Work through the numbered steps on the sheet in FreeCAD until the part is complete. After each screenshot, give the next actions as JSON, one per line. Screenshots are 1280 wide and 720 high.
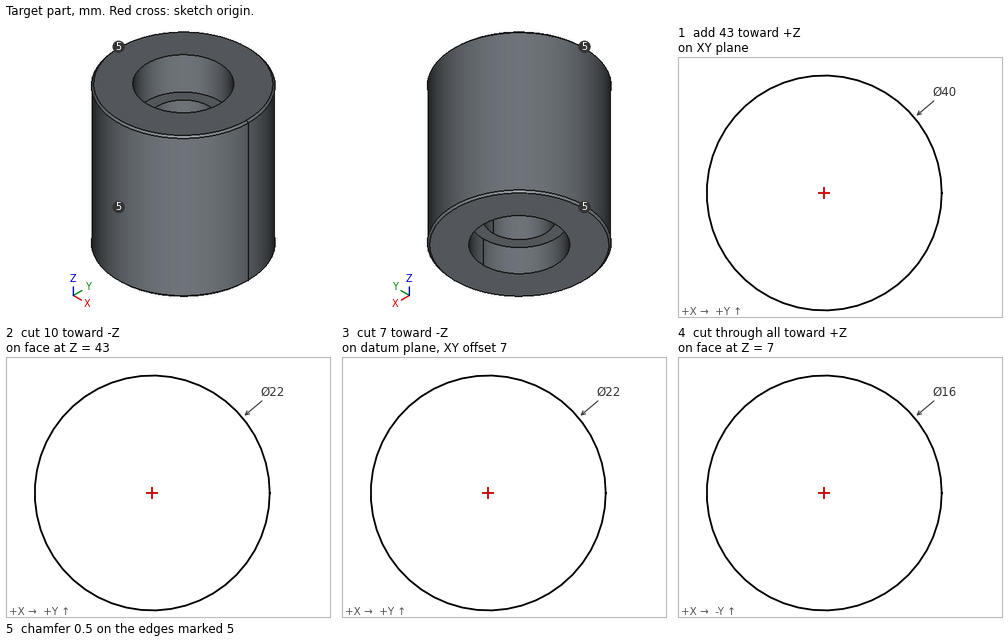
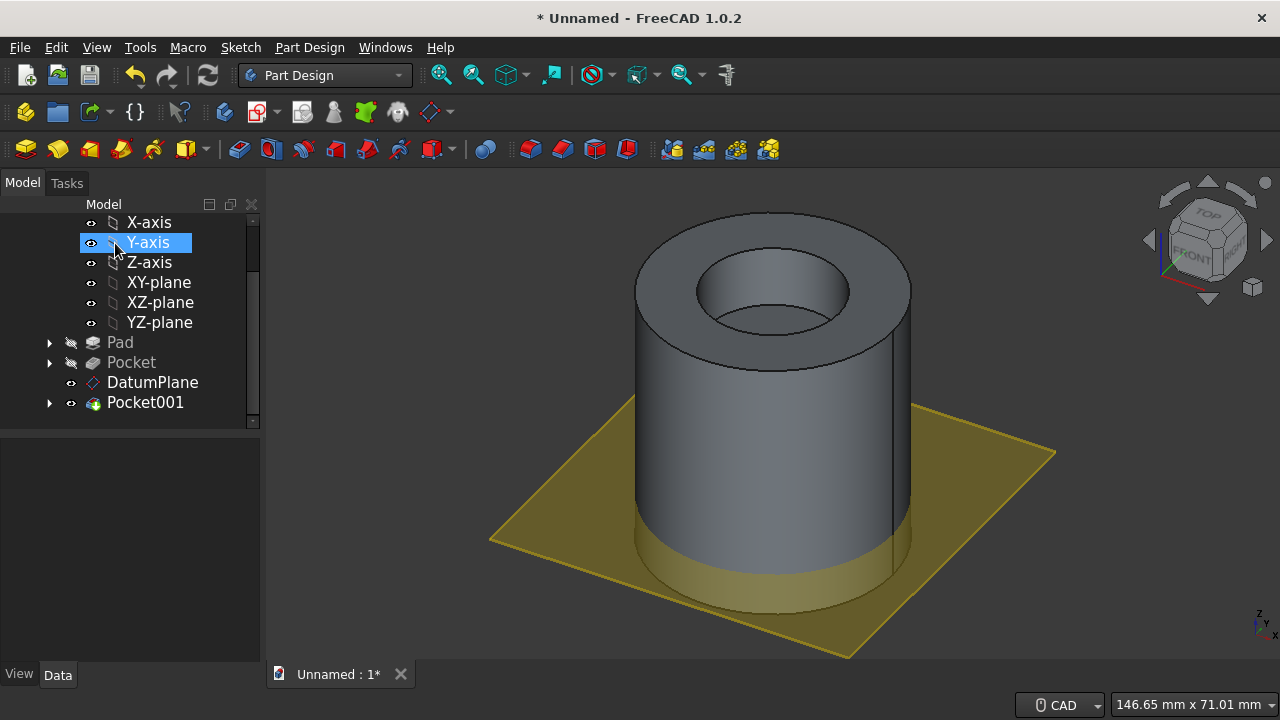
{"action": "left_click", "coordinate": [116, 383]}
{"action": "key", "text": "space"}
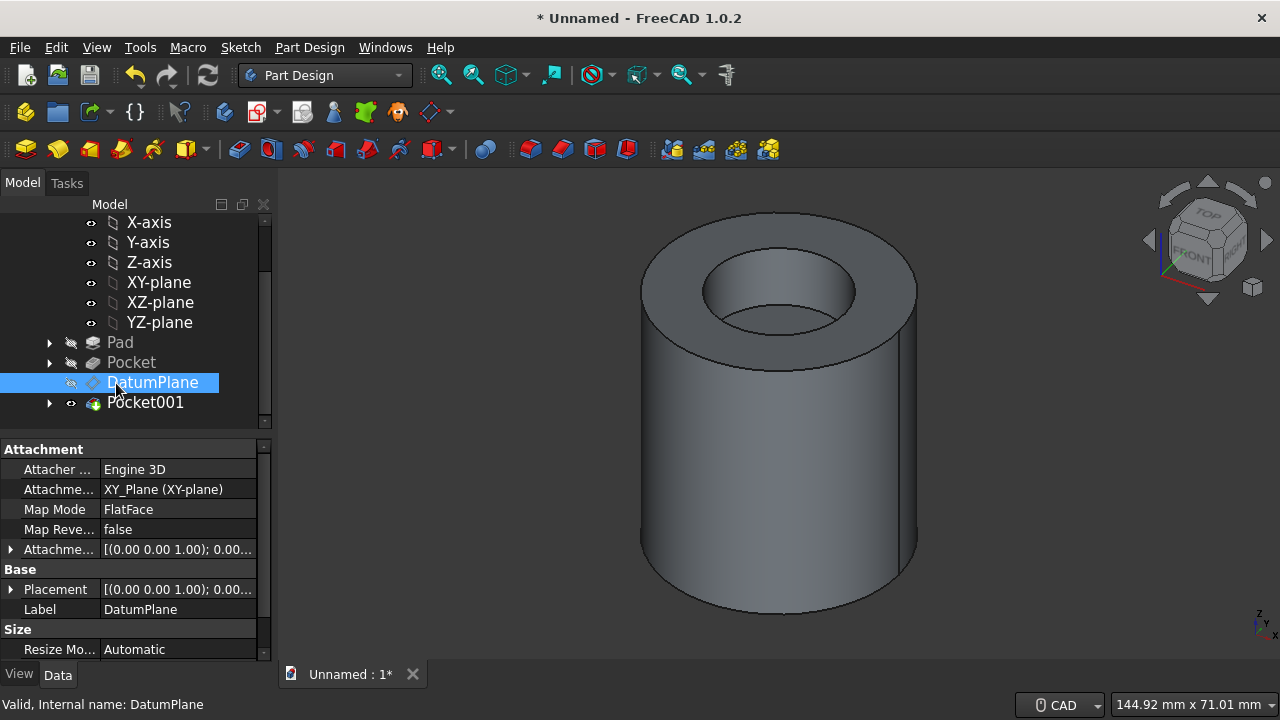
{"action": "key", "text": "5"}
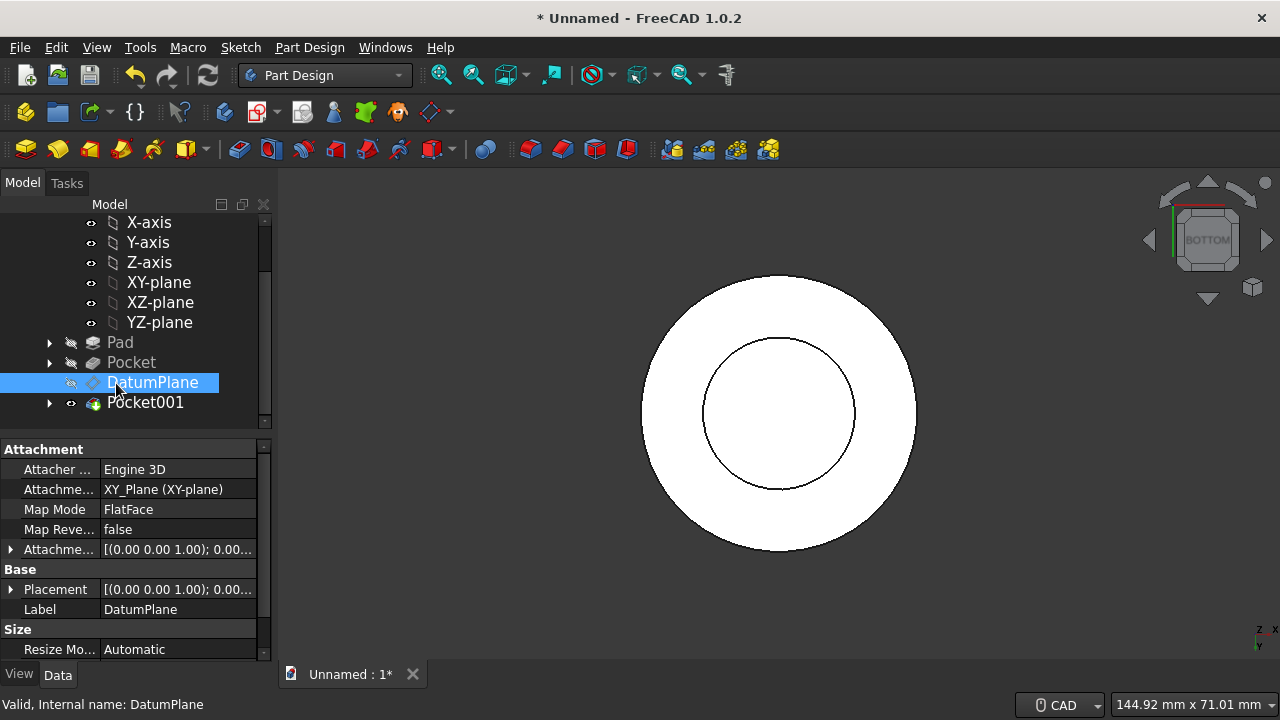
{"action": "left_click", "coordinate": [779, 412]}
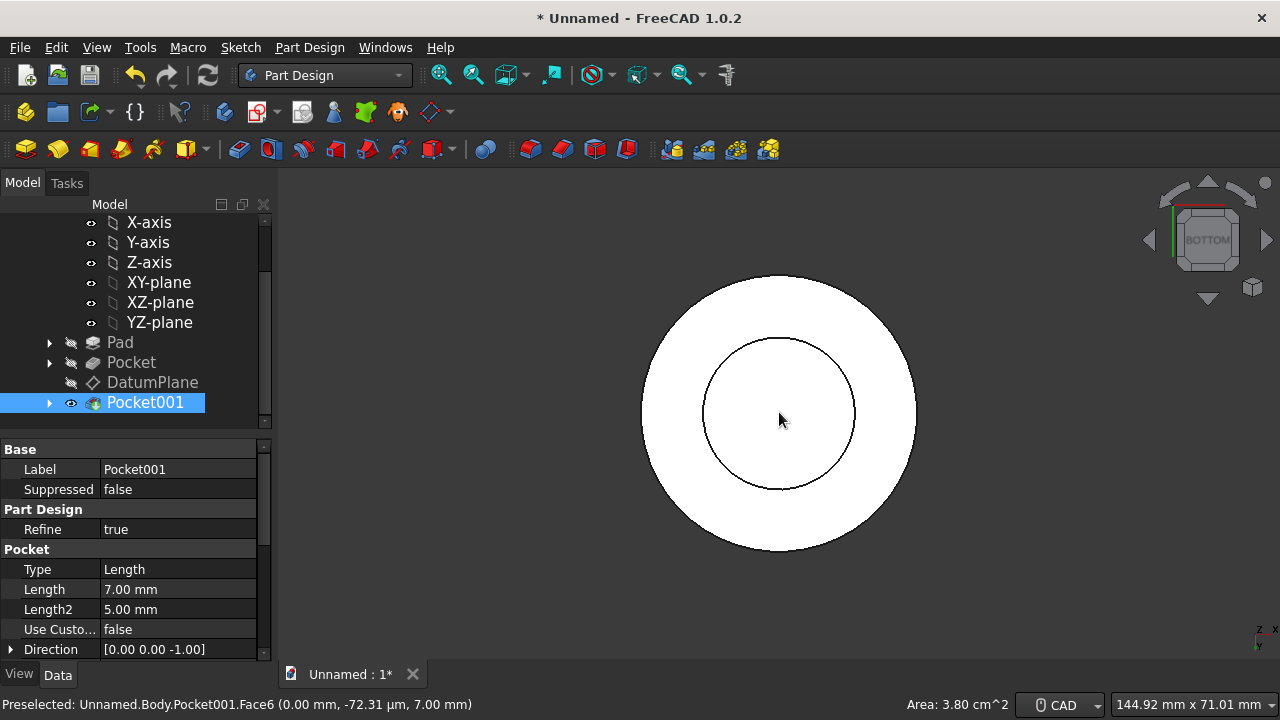
{"action": "left_click", "coordinate": [258, 112]}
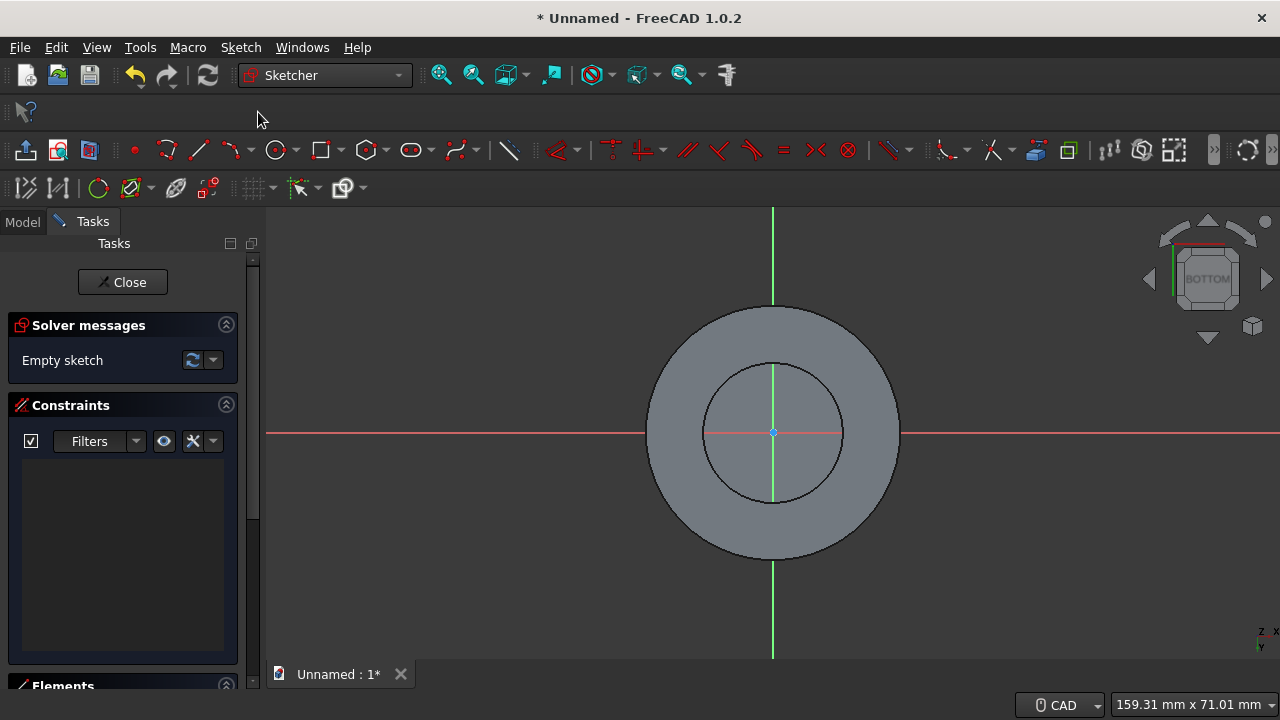
{"action": "left_click", "coordinate": [90, 150]}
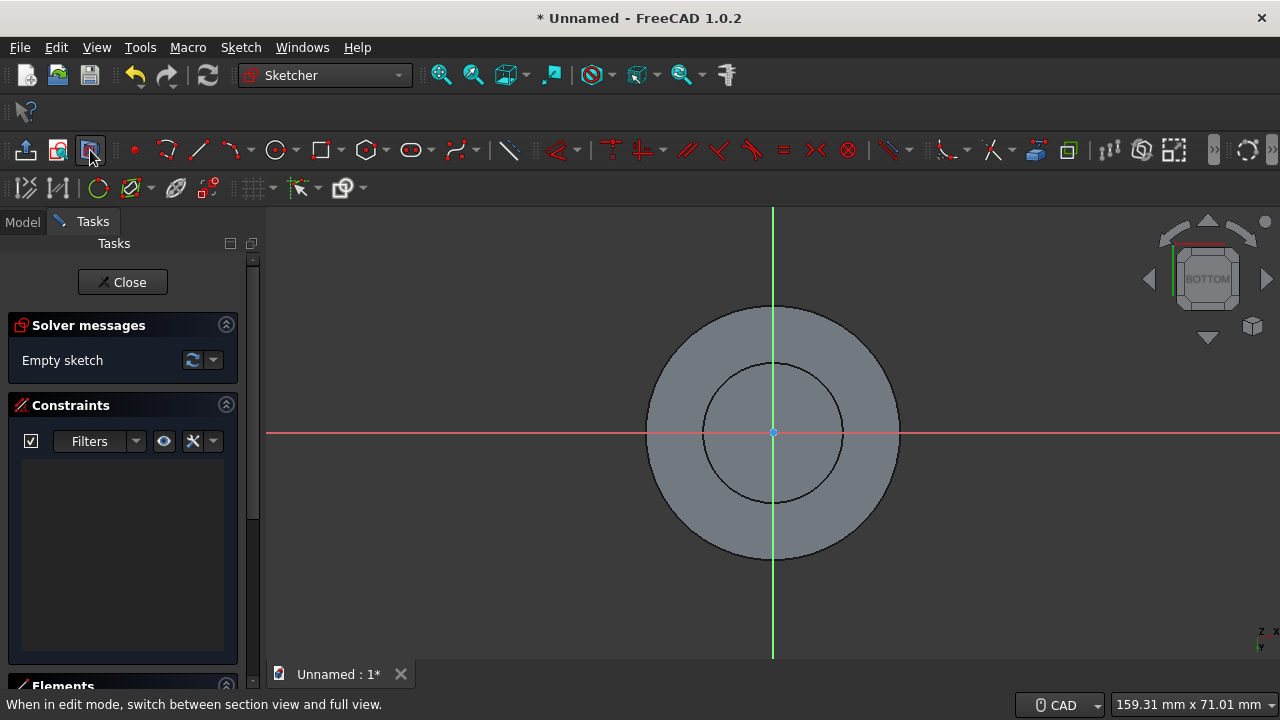
{"action": "scroll", "coordinate": [813, 433], "scroll_direction": "up", "scroll_amount": 5}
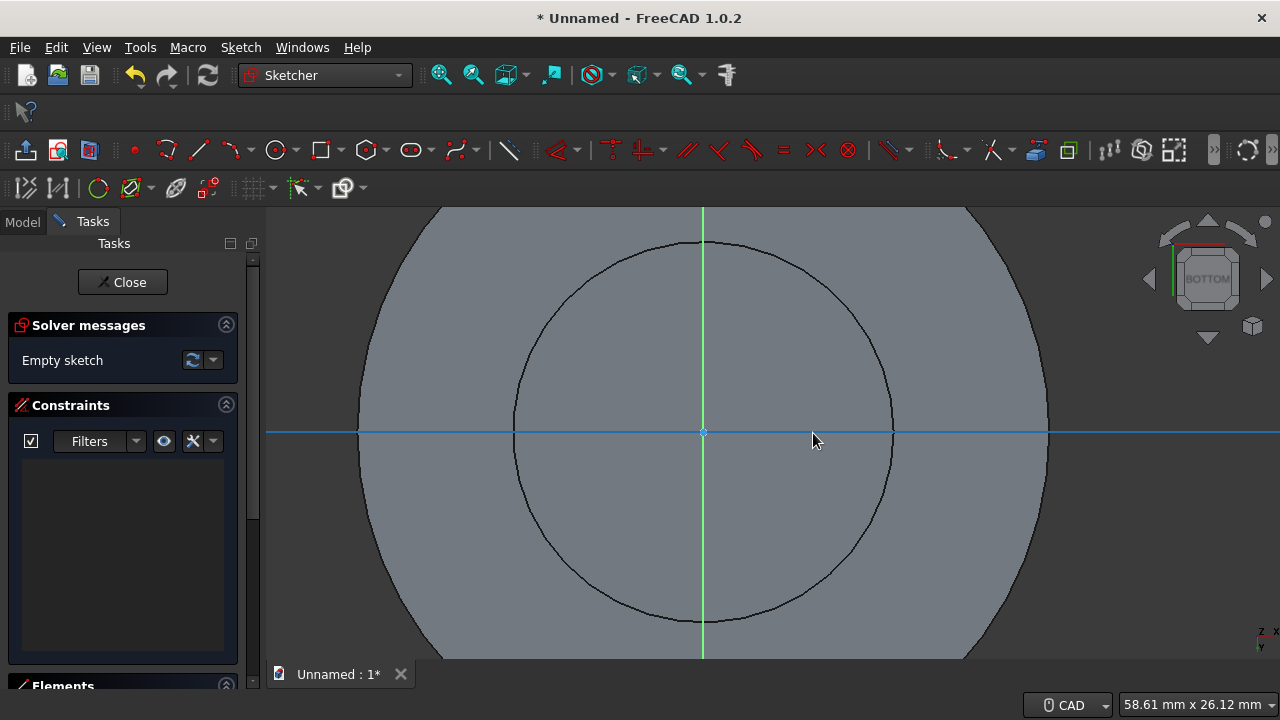
{"action": "left_click", "coordinate": [276, 150]}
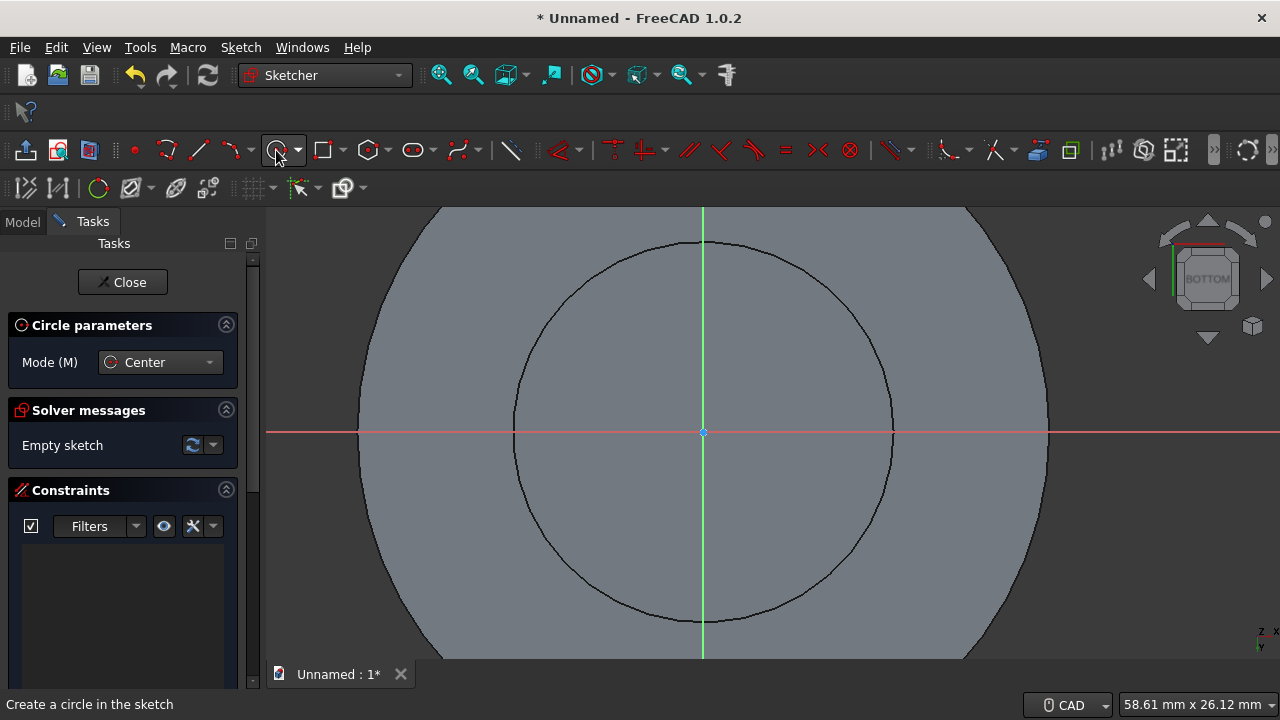
{"action": "left_click", "coordinate": [703, 432]}
{"action": "mouse_move", "coordinate": [801, 334]}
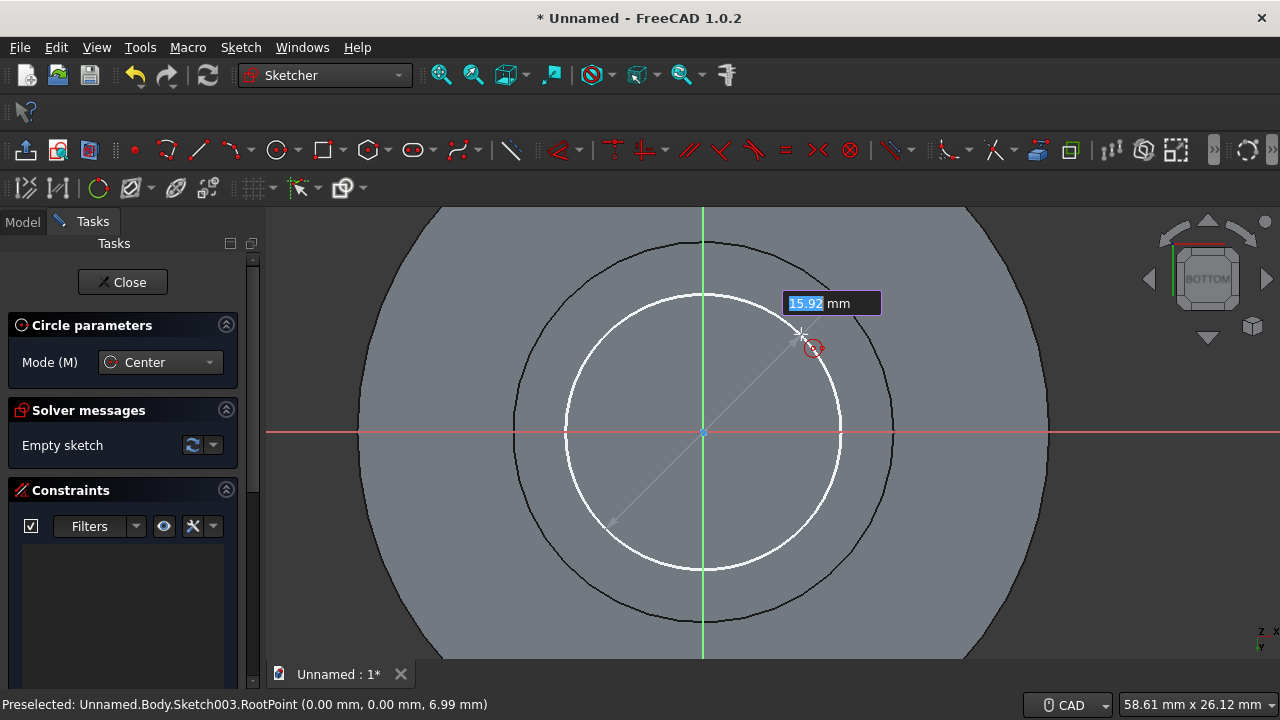
{"action": "type", "text": "16"}
{"action": "key", "text": "Return"}
{"action": "key", "text": "Escape"}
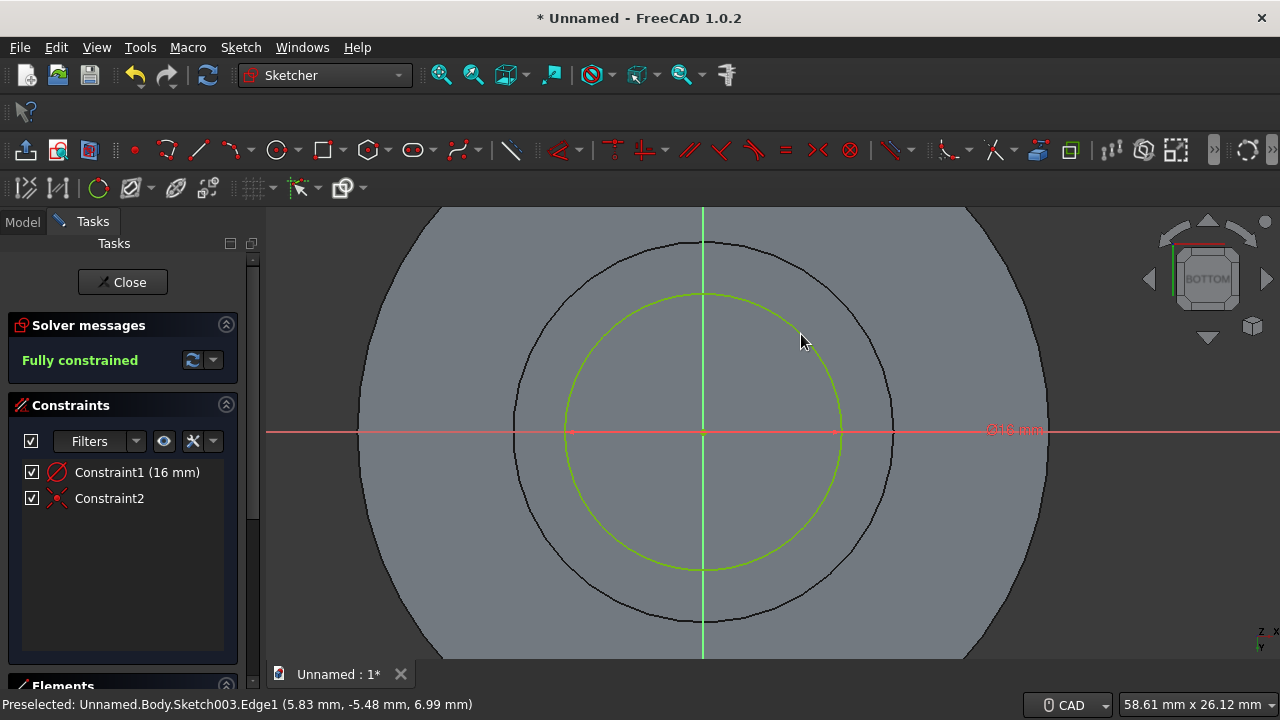
{"action": "left_click", "coordinate": [123, 282]}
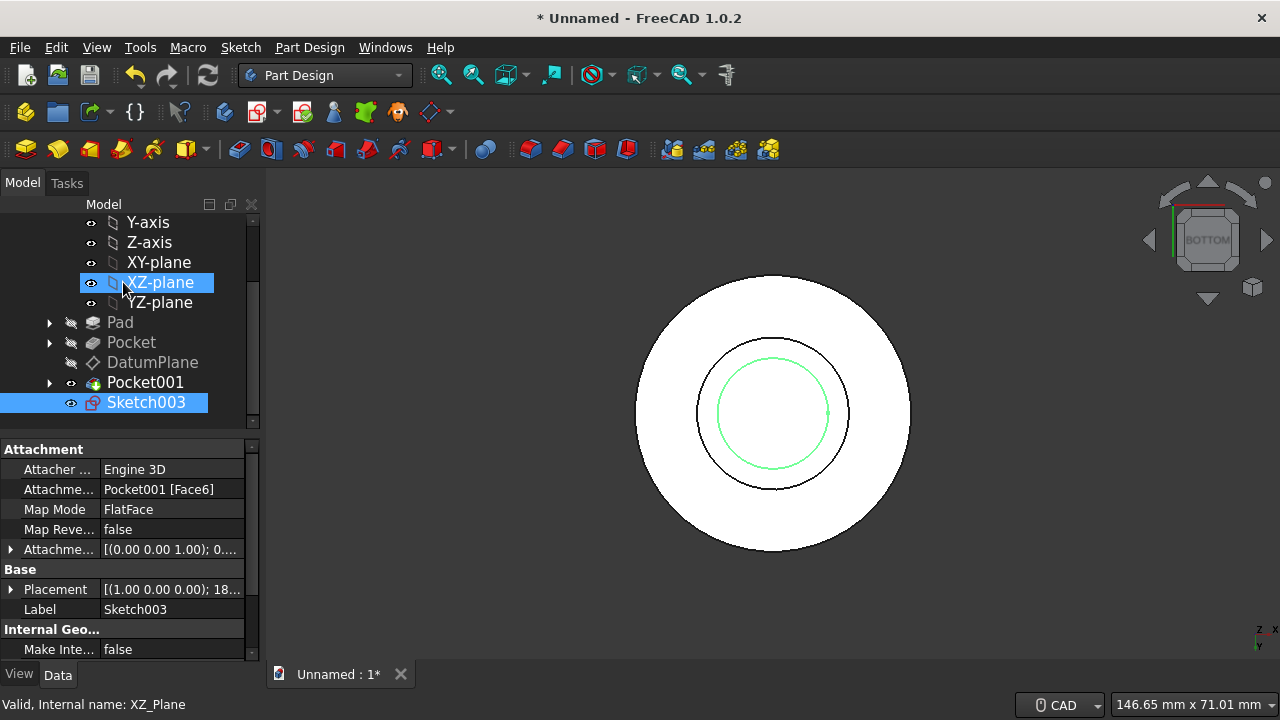
{"action": "left_click", "coordinate": [240, 150]}